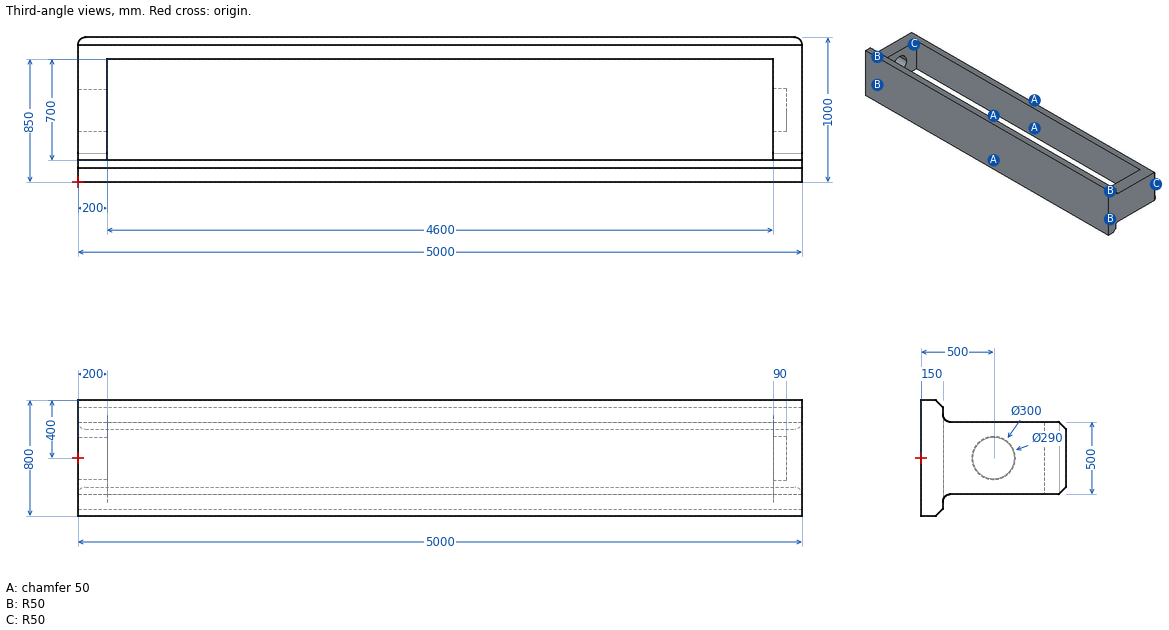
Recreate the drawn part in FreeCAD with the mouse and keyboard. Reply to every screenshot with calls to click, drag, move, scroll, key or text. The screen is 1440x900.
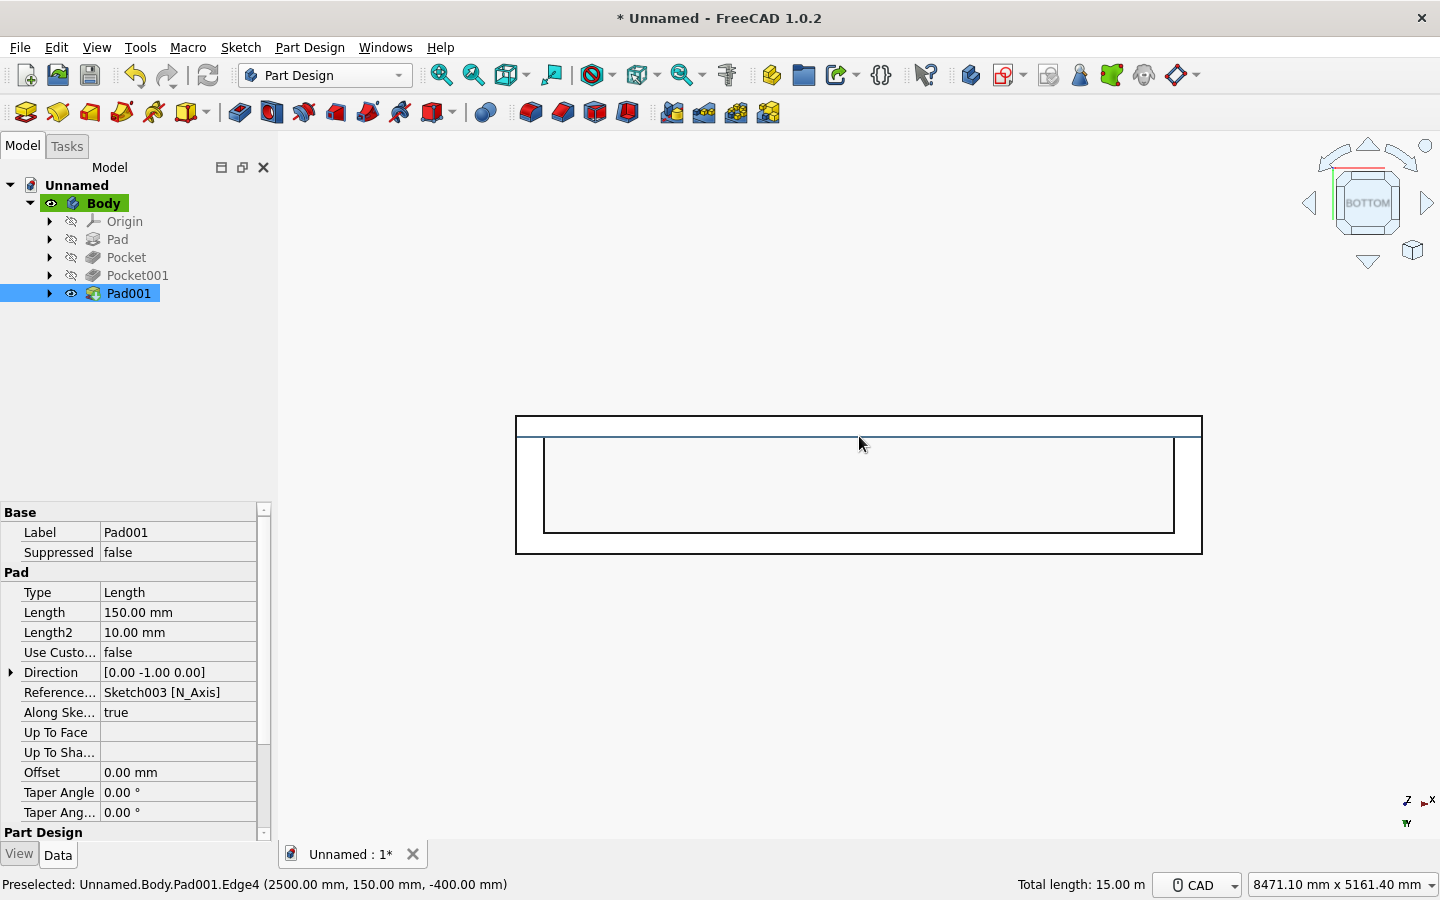
click(859, 553, ctrl)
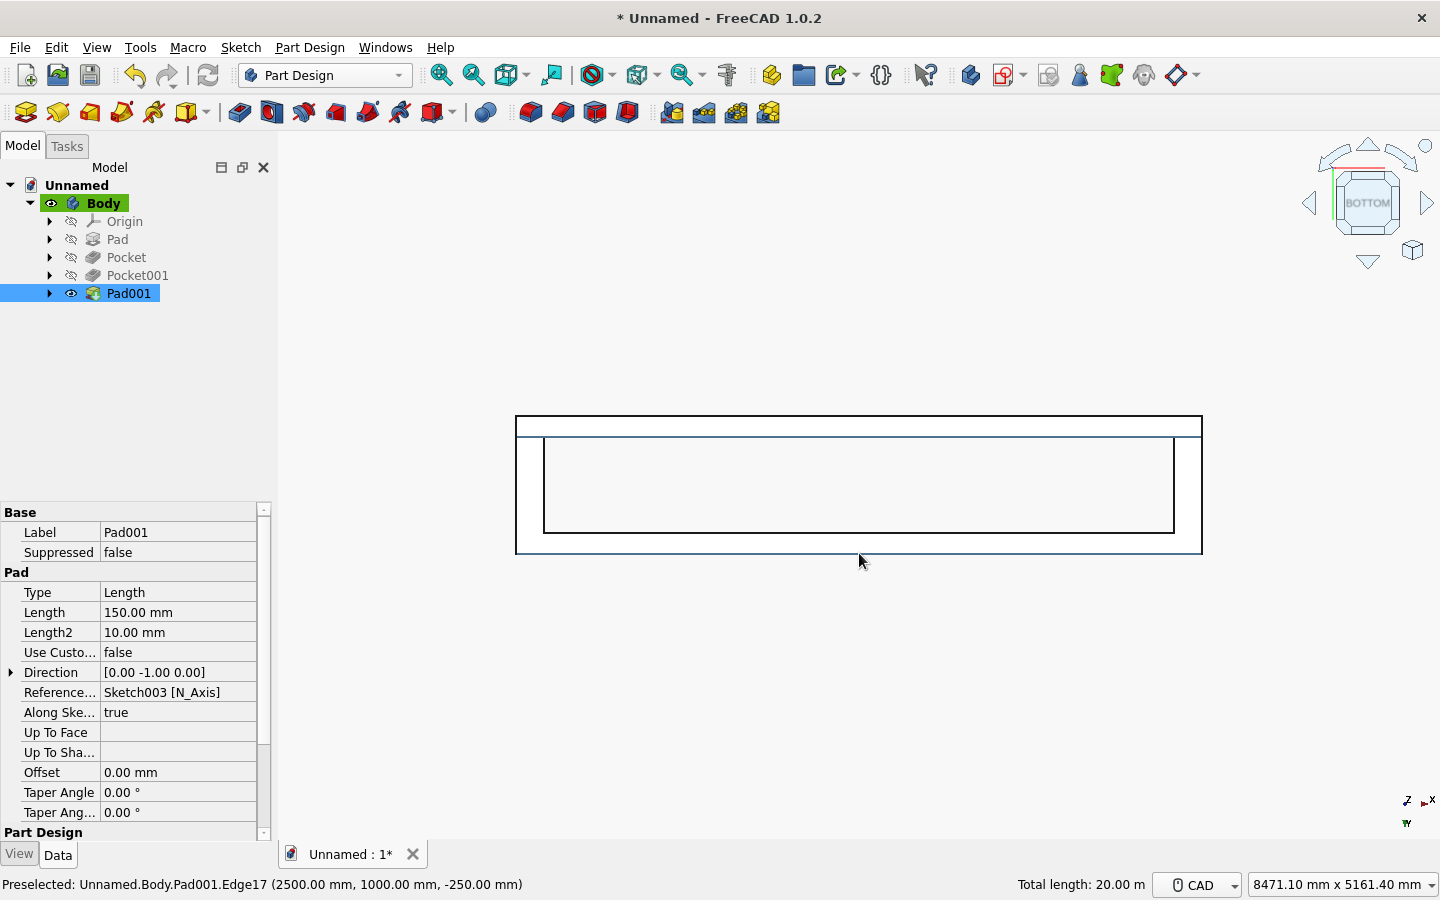
click(564, 112)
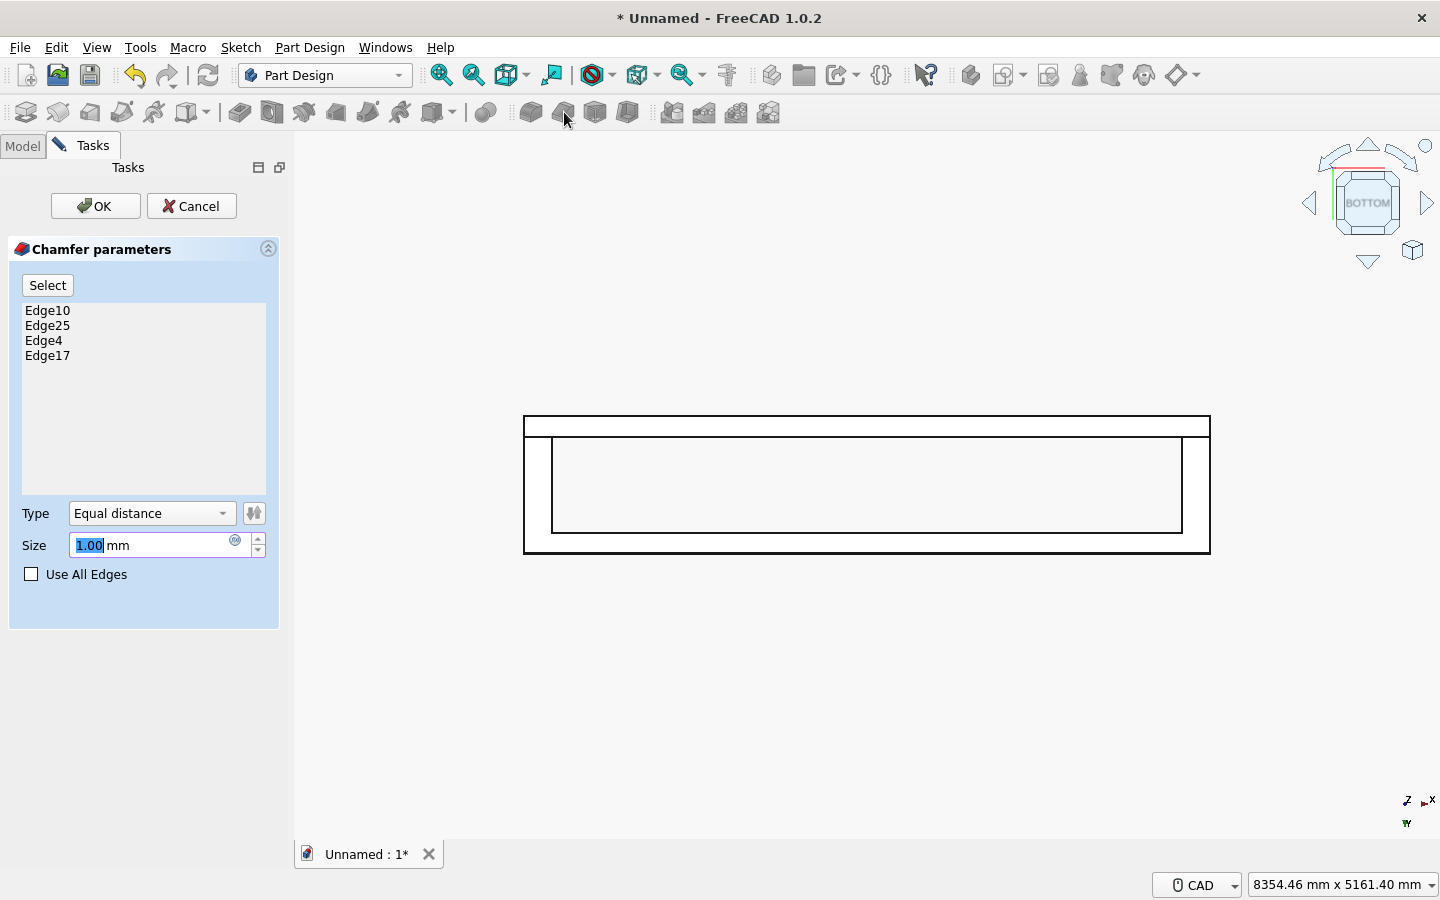
text(50)
key(Tab)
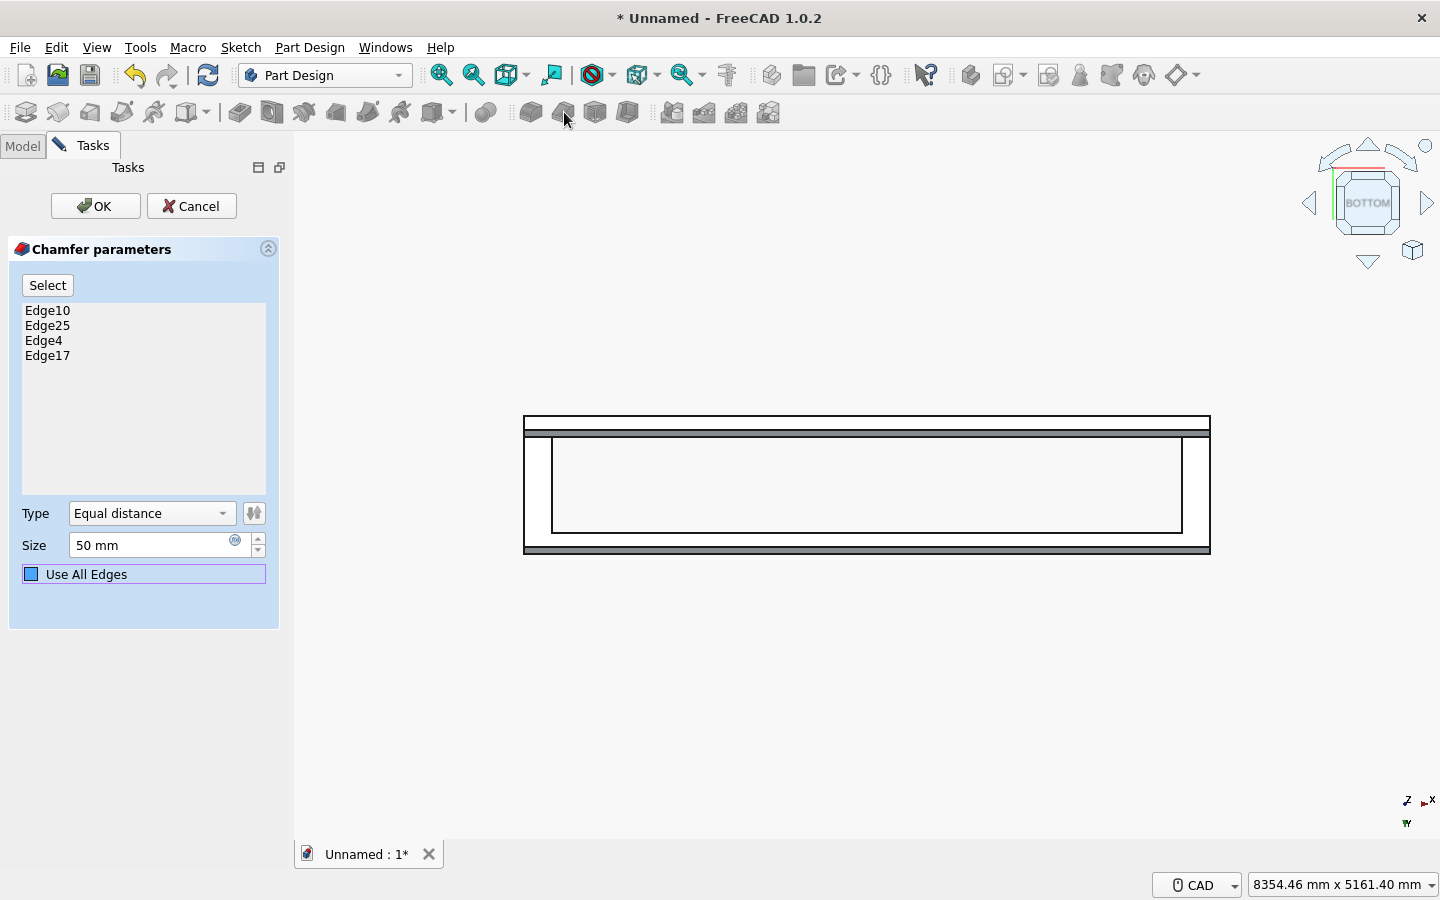
click(96, 206)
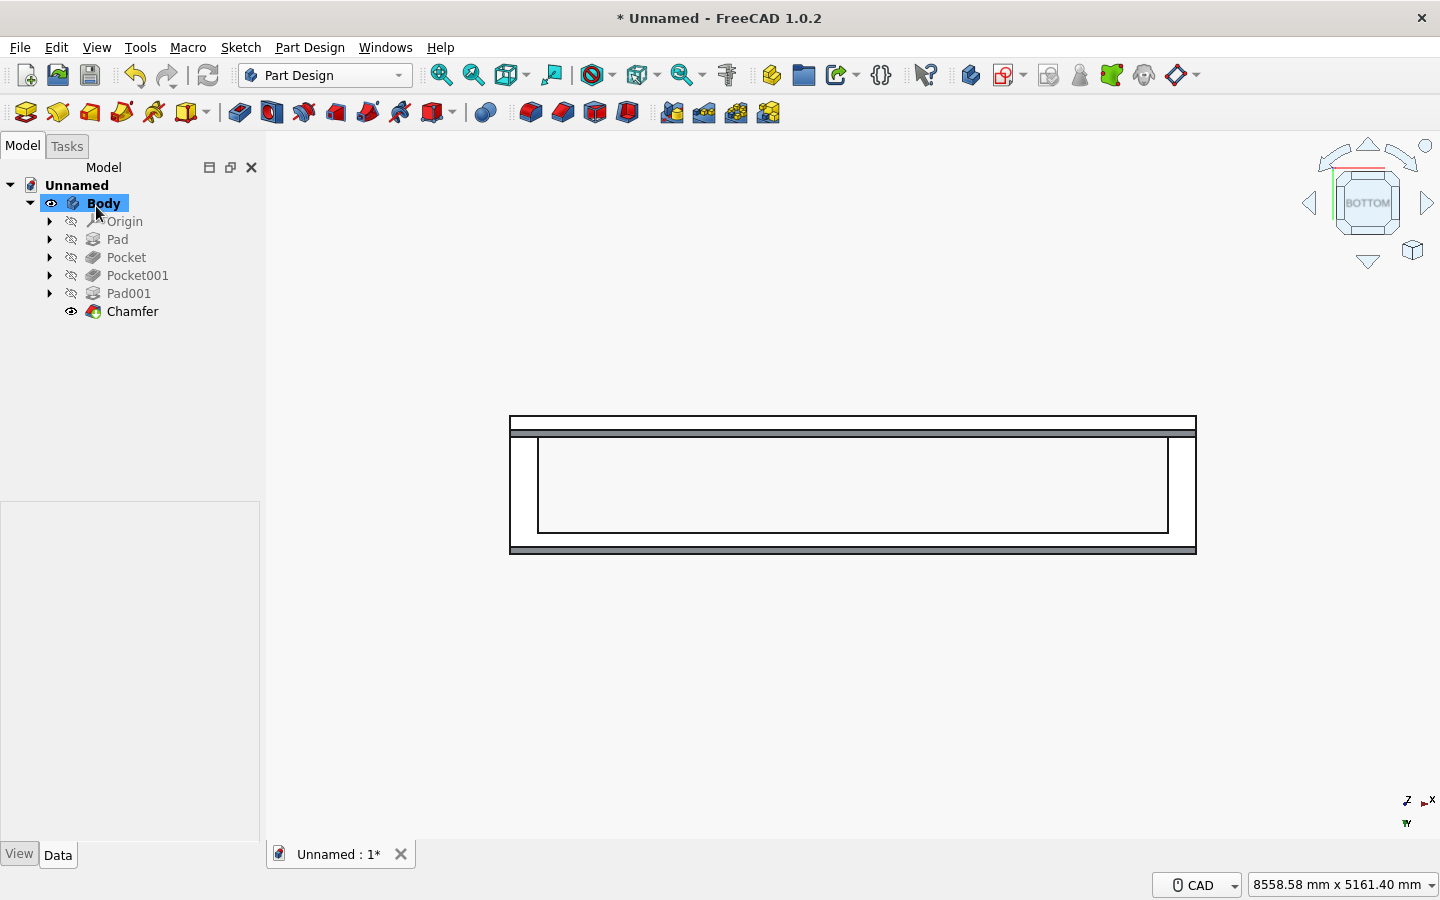
key(0)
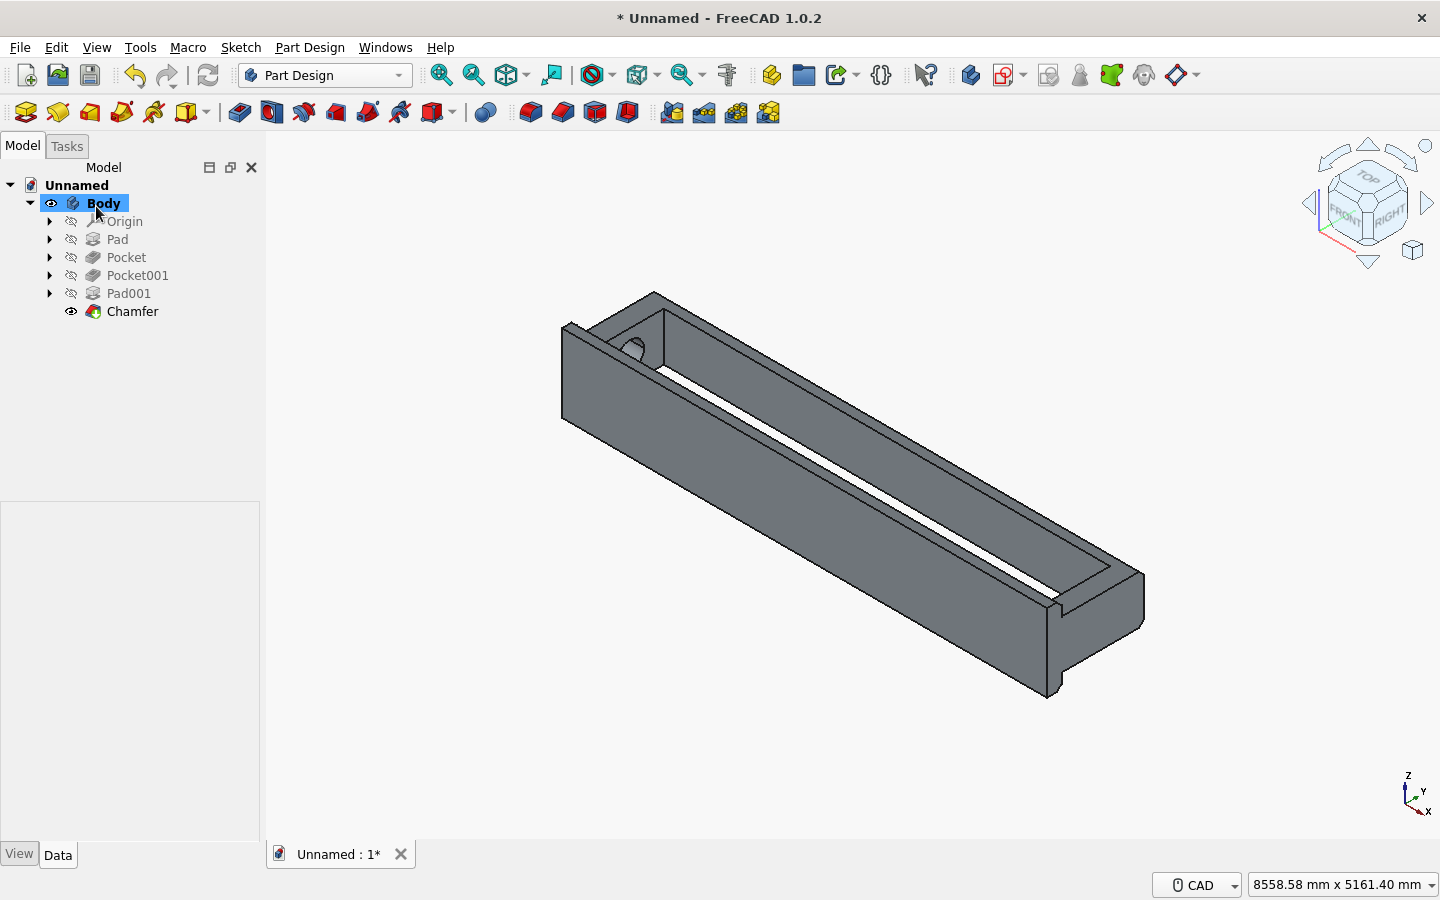
key(2)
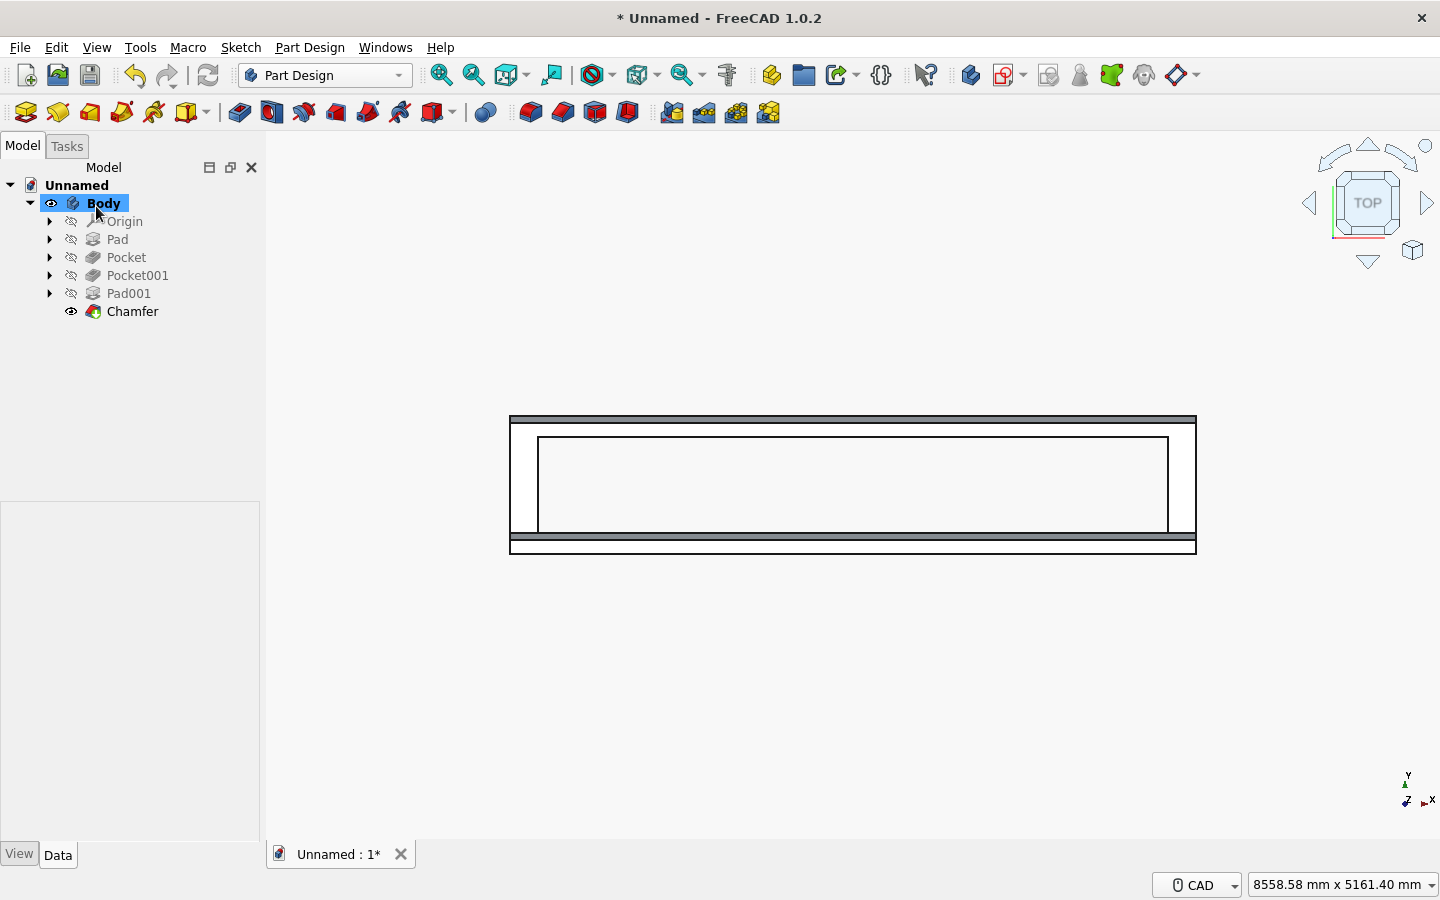
key(1)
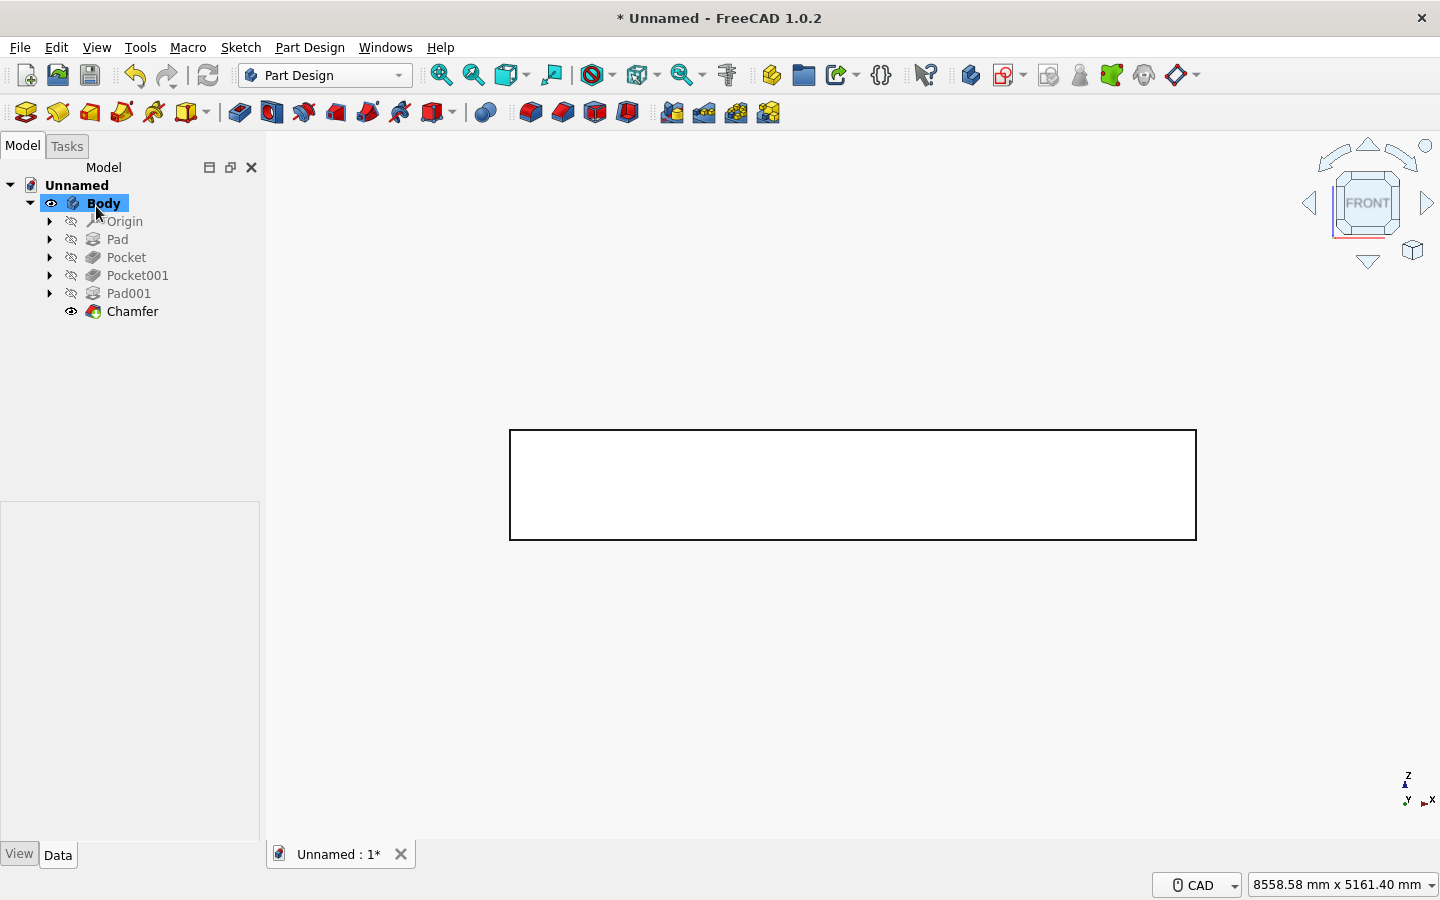
key(3)